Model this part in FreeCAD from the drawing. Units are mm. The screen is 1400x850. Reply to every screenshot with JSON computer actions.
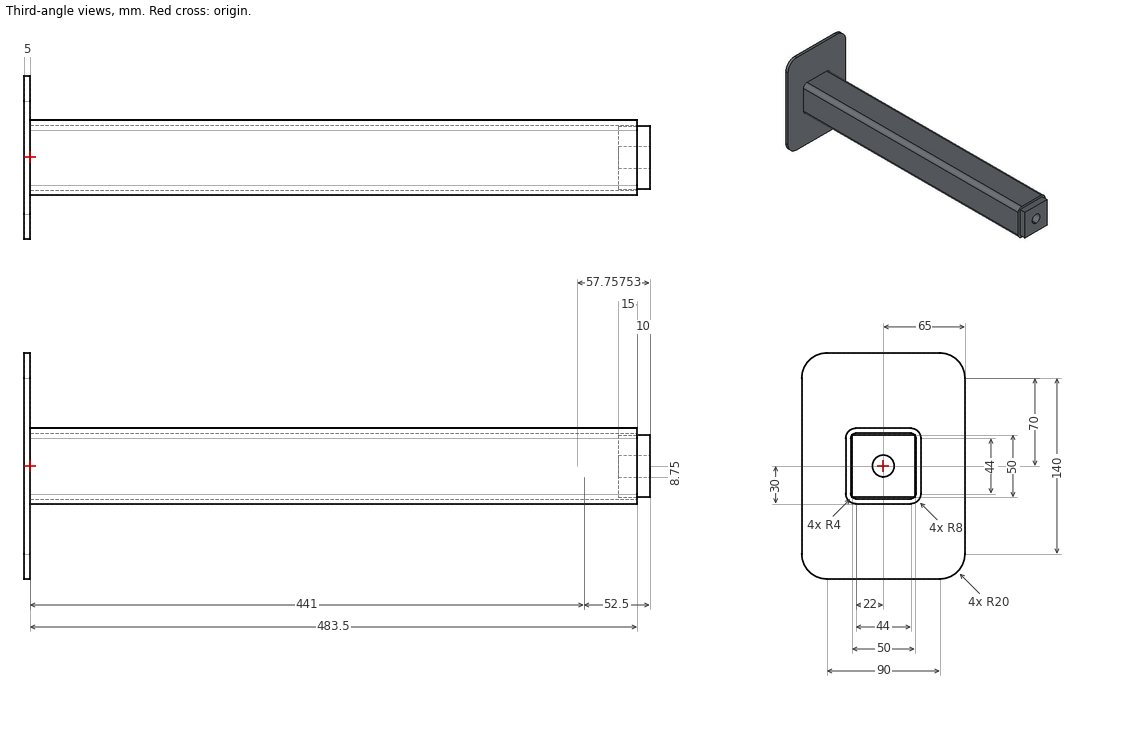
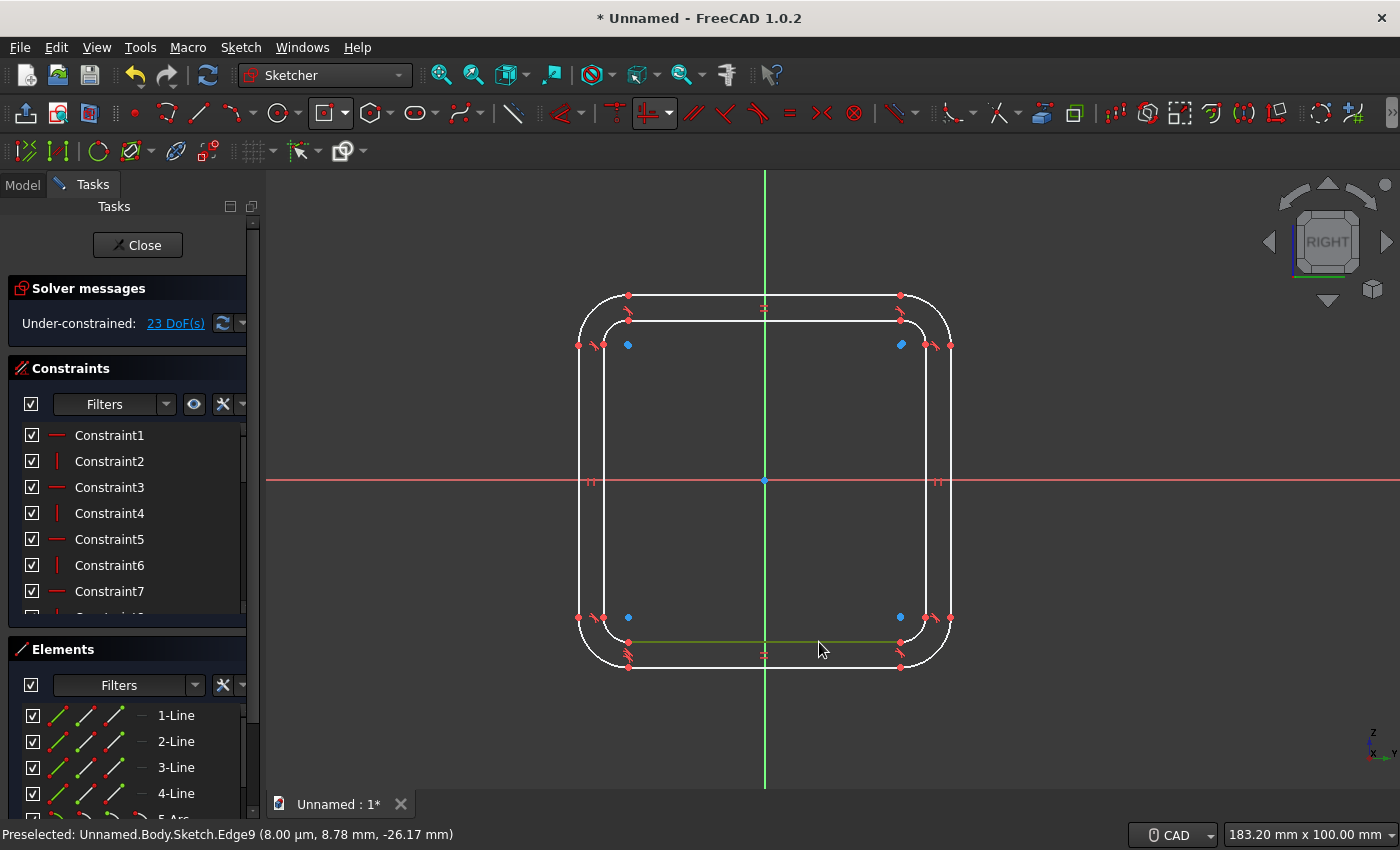
{"action": "left_click", "coordinate": [912, 639]}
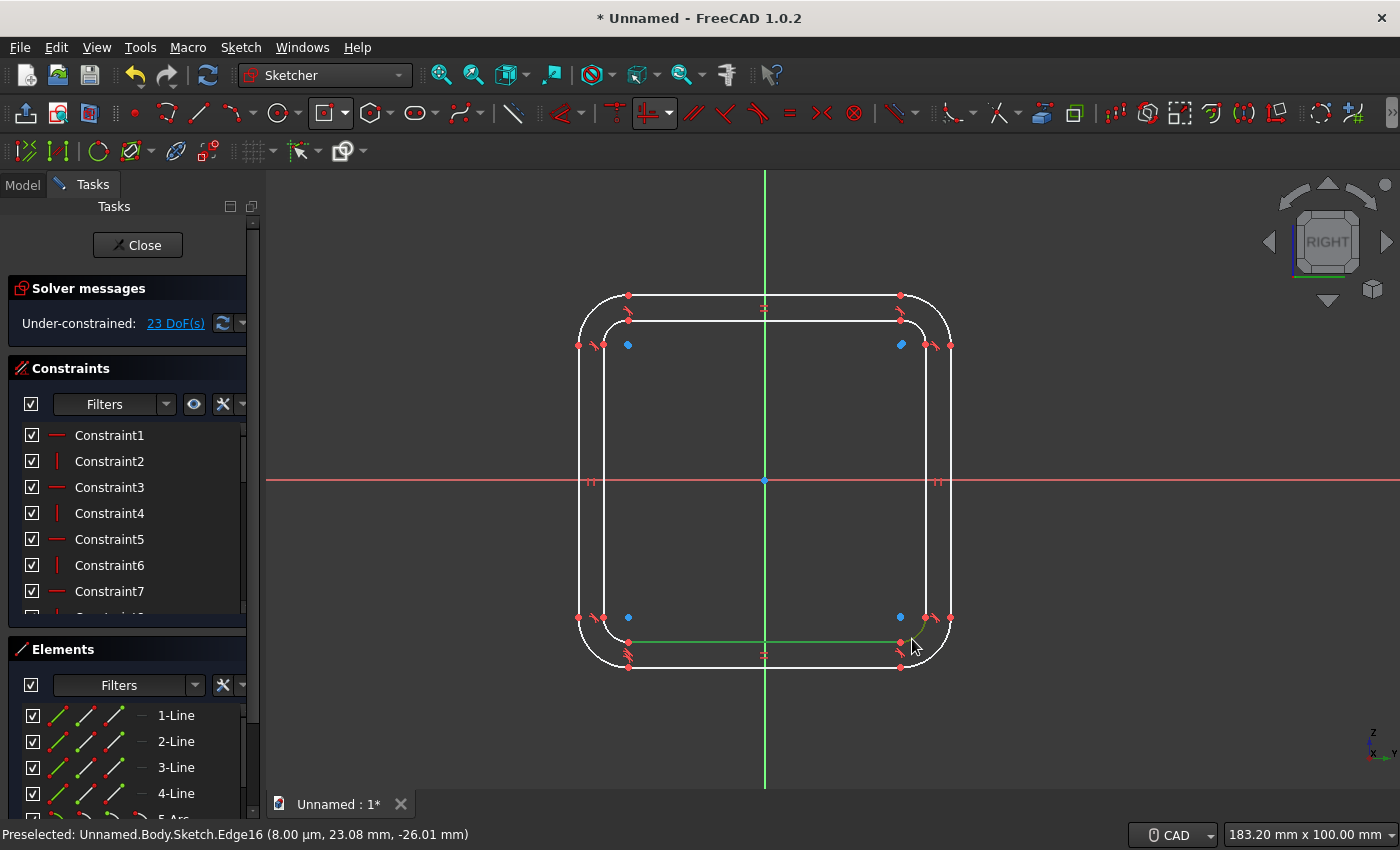
{"action": "left_click", "coordinate": [758, 114]}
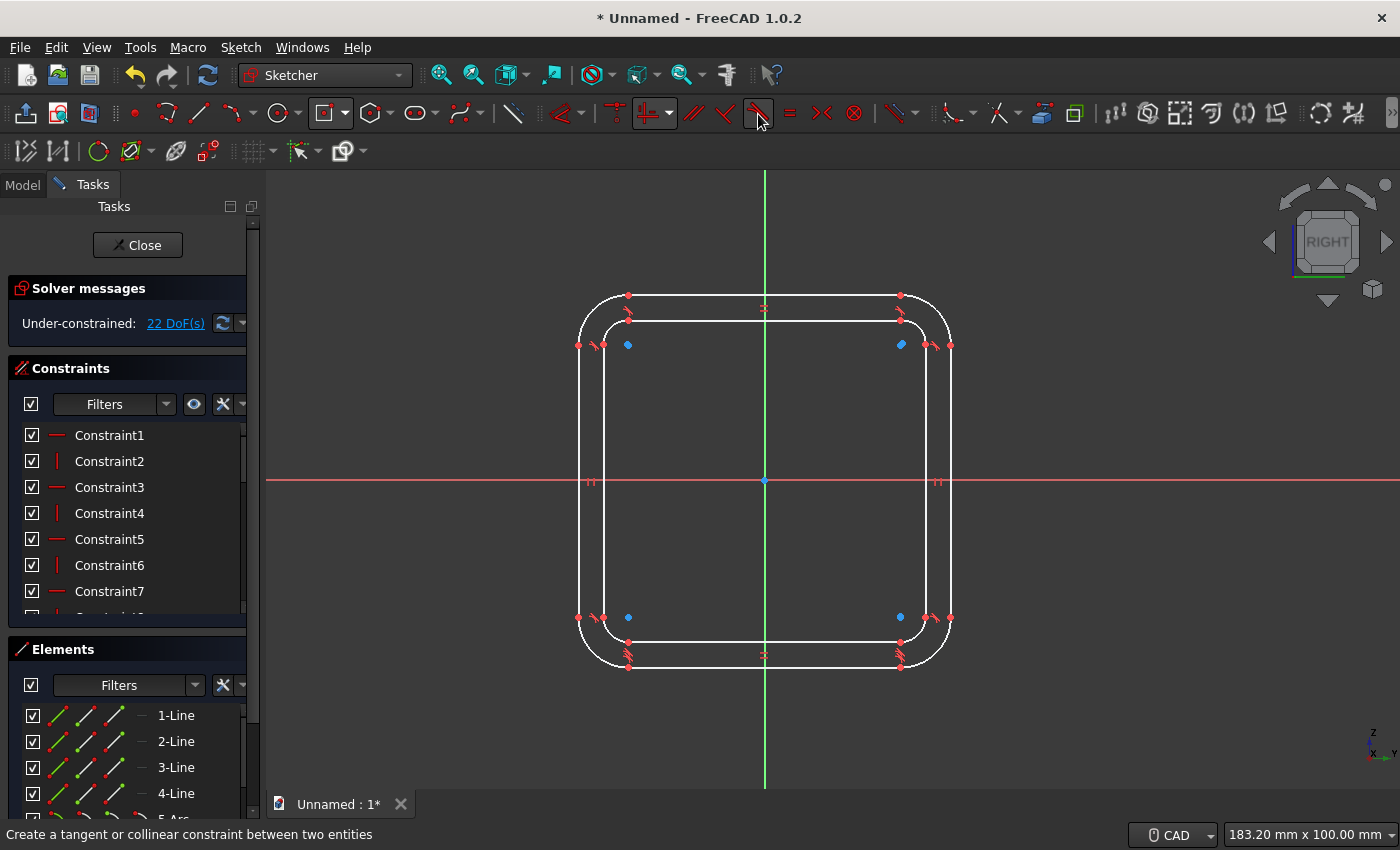
{"action": "left_click", "coordinate": [604, 536]}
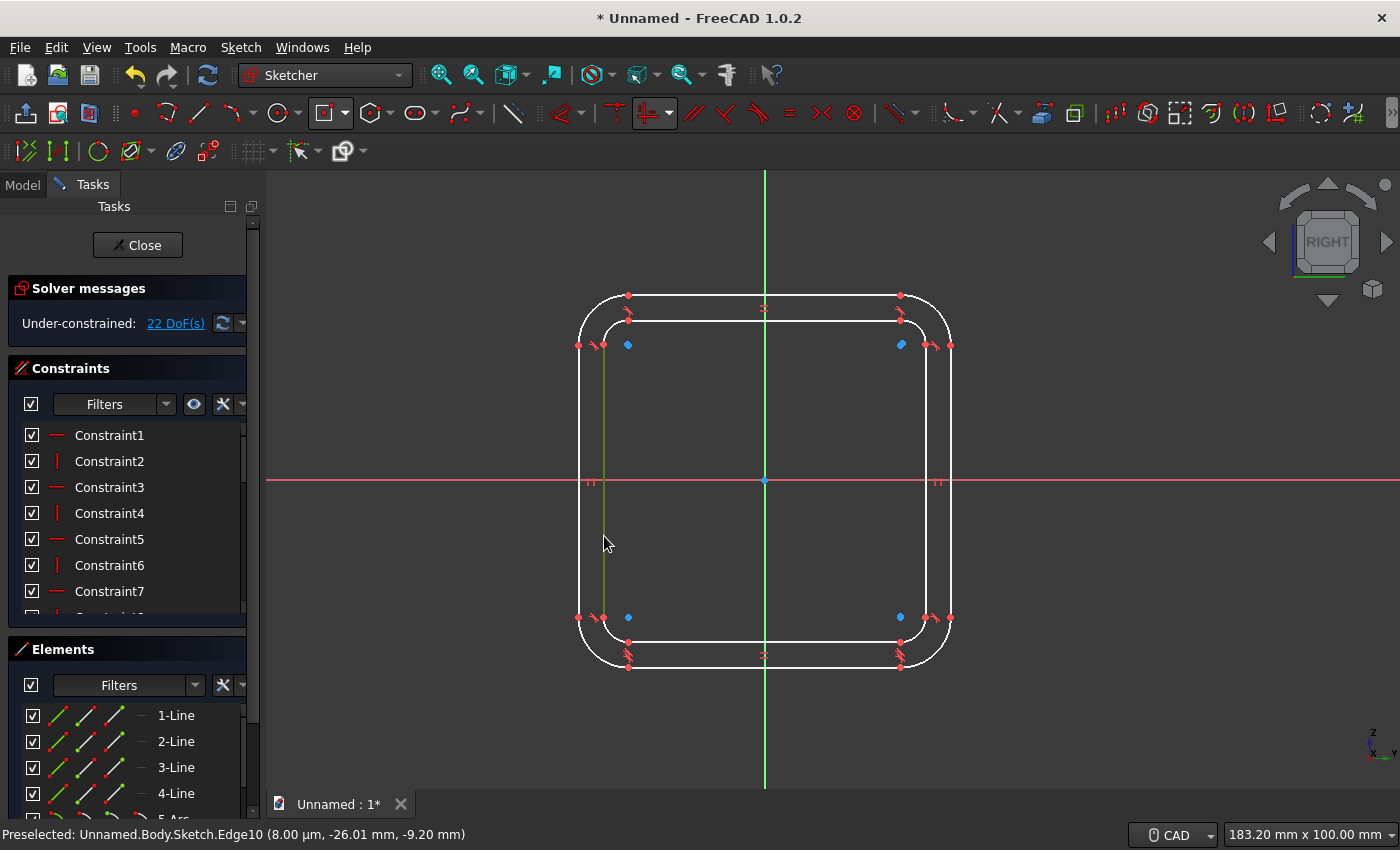
{"action": "left_click", "coordinate": [607, 629]}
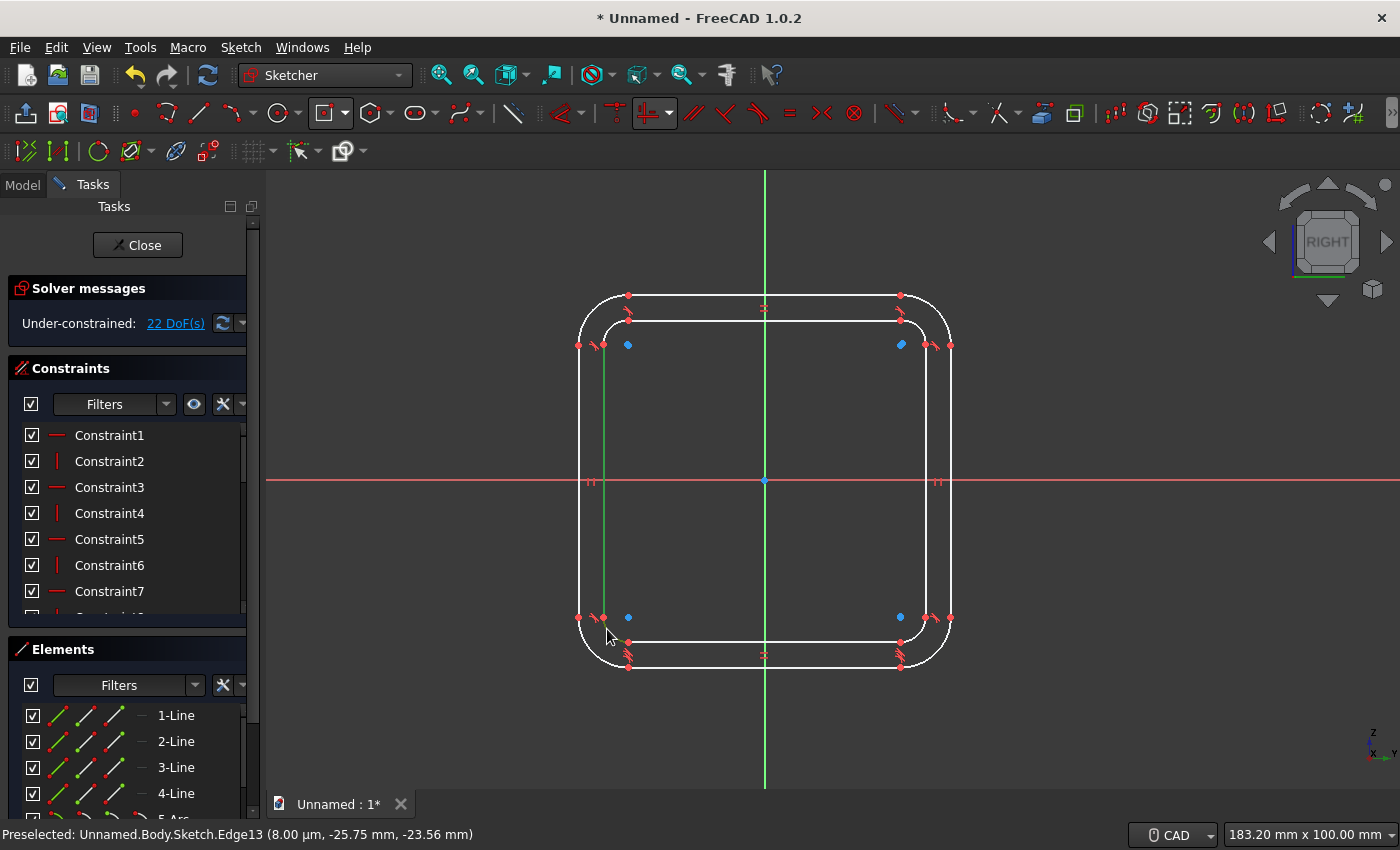
{"action": "left_click", "coordinate": [758, 114]}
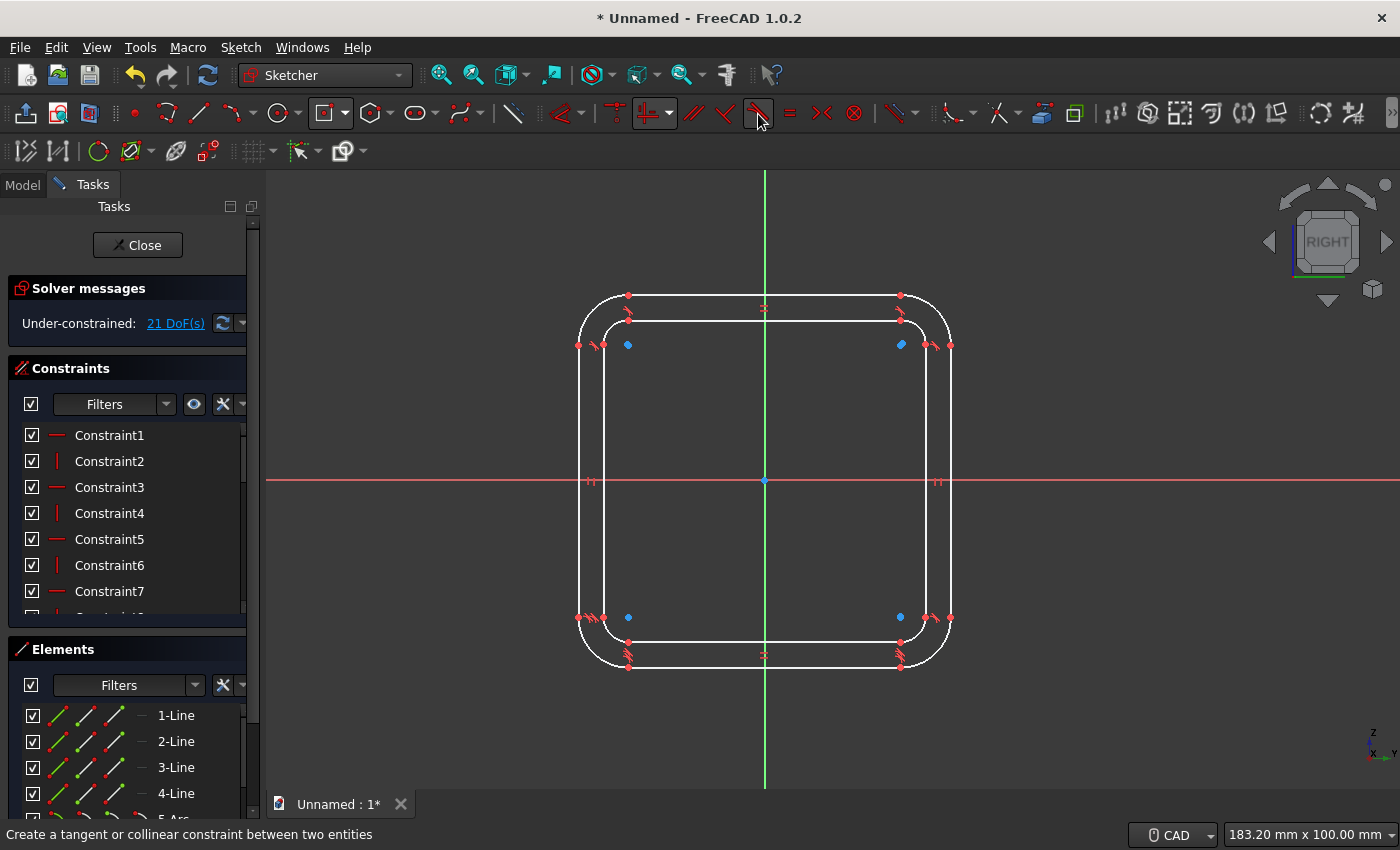
{"action": "left_click", "coordinate": [604, 535]}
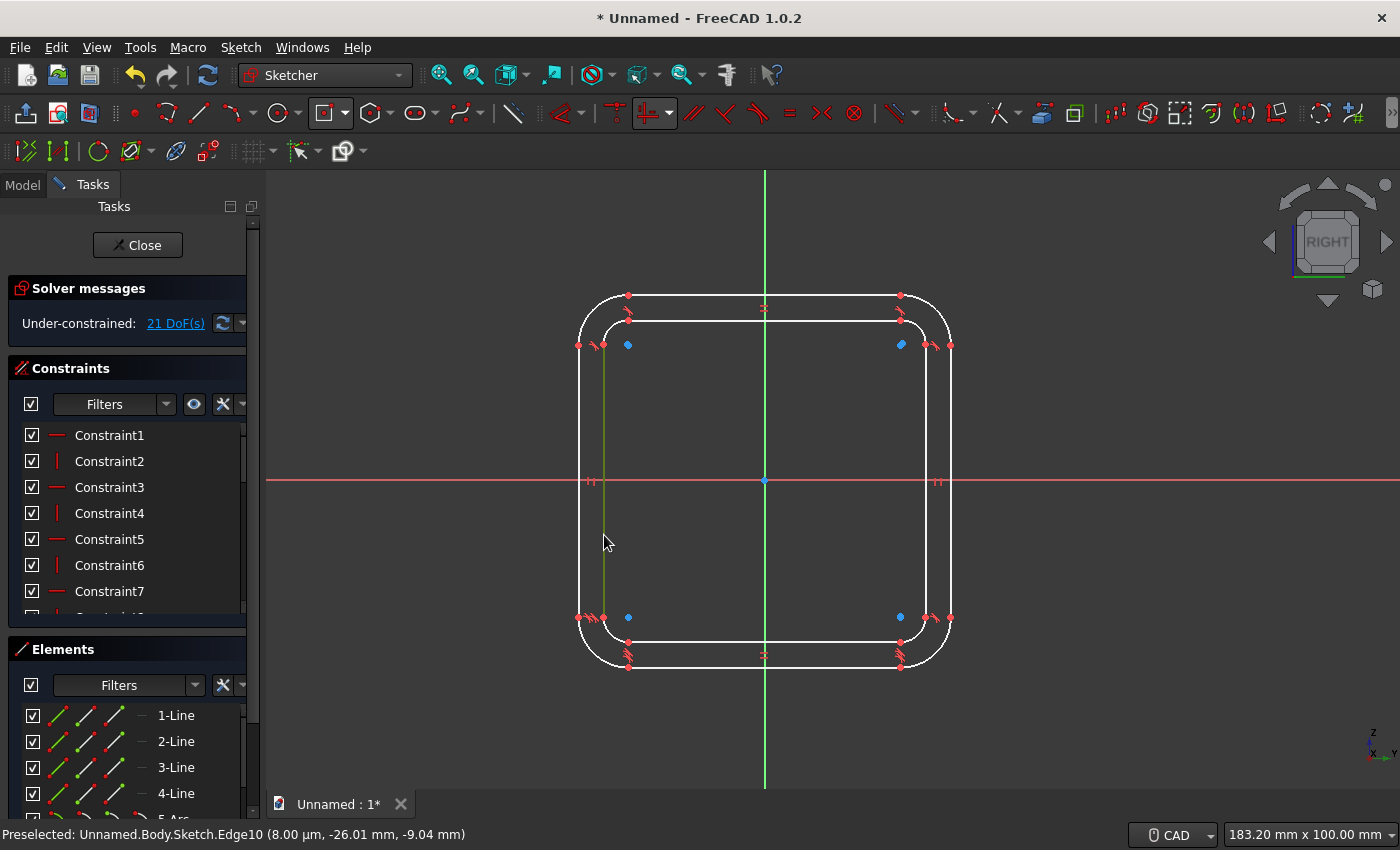
{"action": "left_click", "coordinate": [617, 323]}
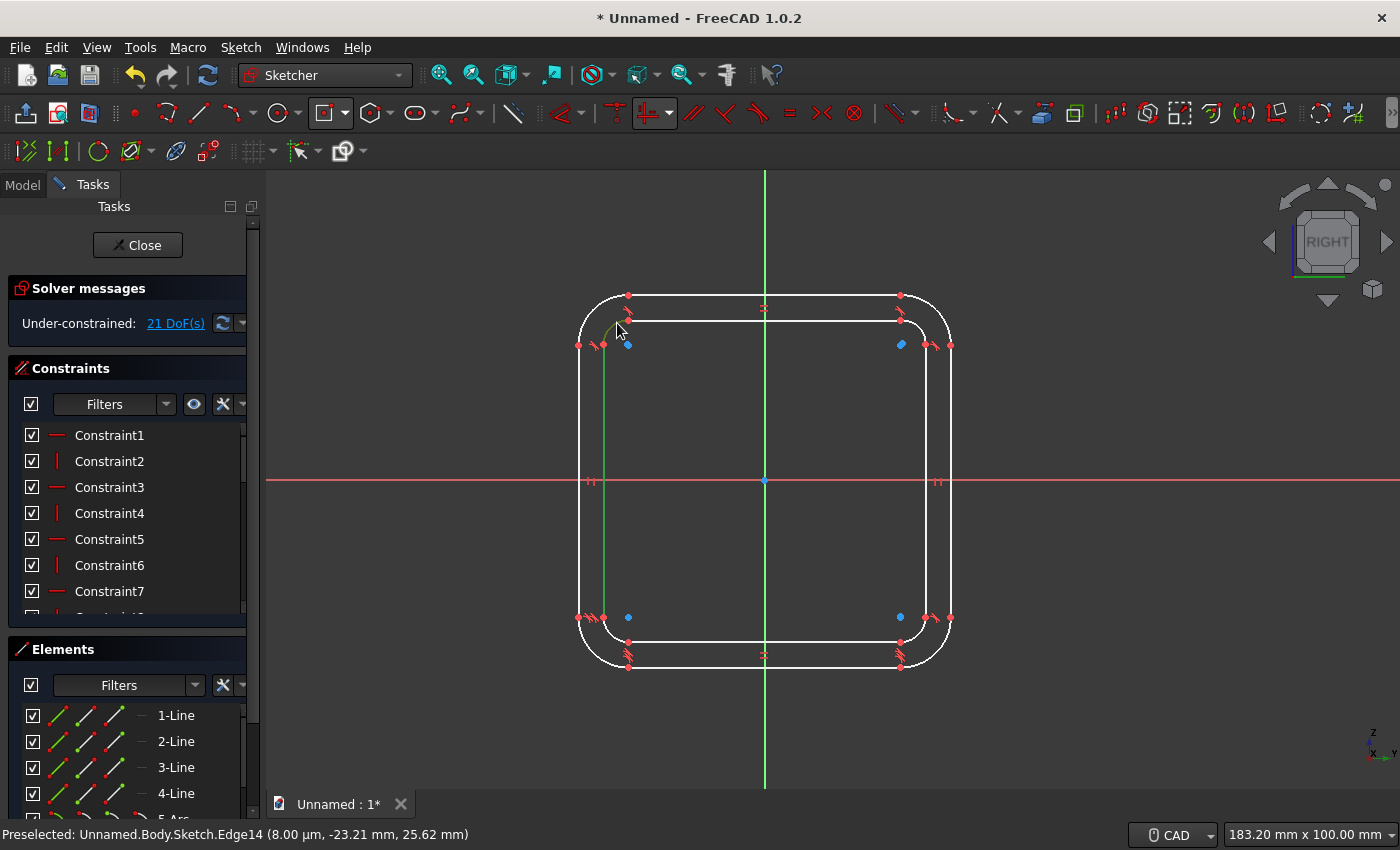
{"action": "left_click", "coordinate": [758, 114]}